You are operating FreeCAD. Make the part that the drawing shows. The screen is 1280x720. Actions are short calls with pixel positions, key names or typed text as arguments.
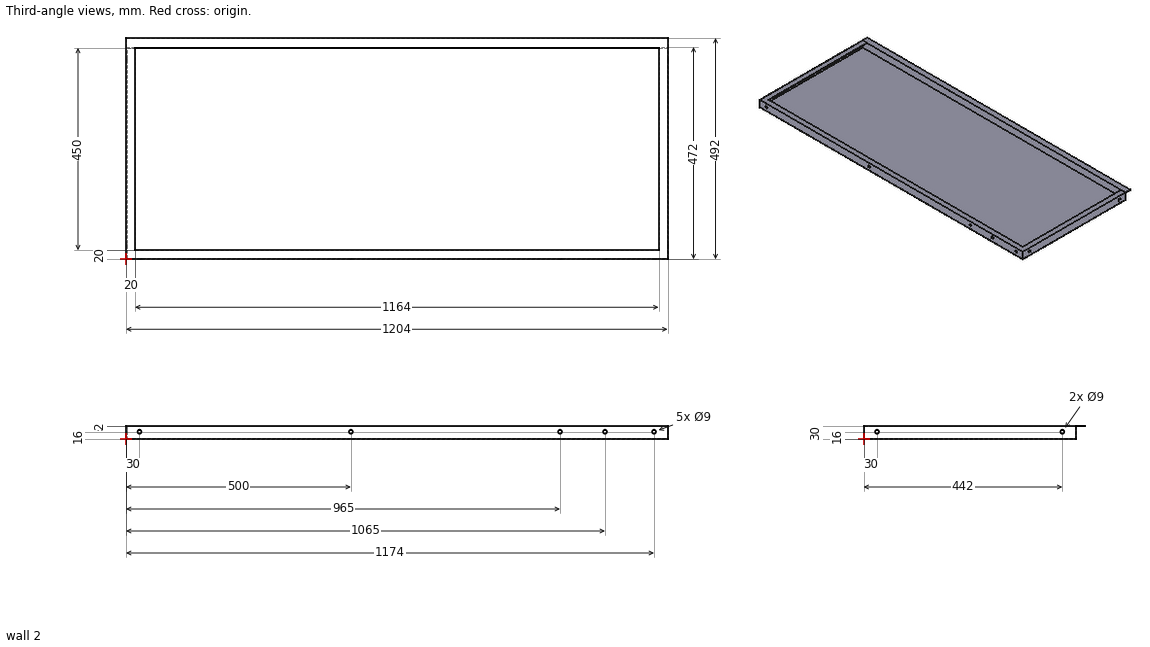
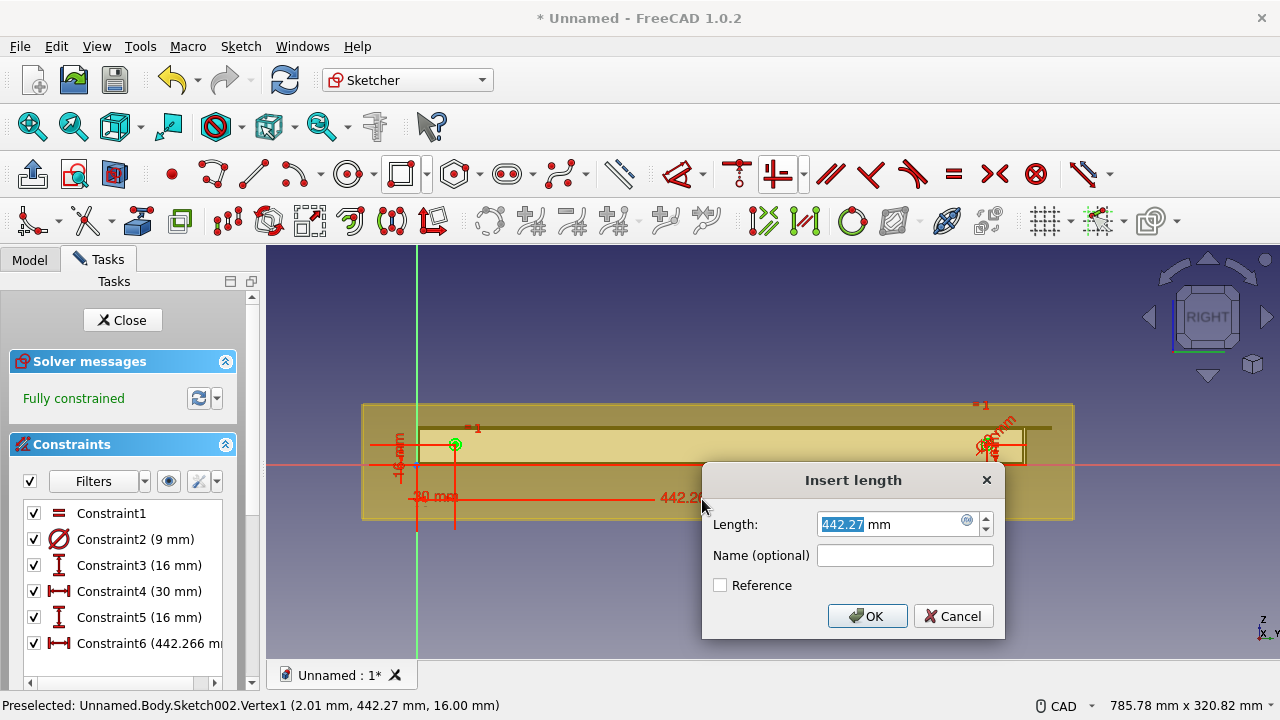
text(442)
key(Return)
key(Escape)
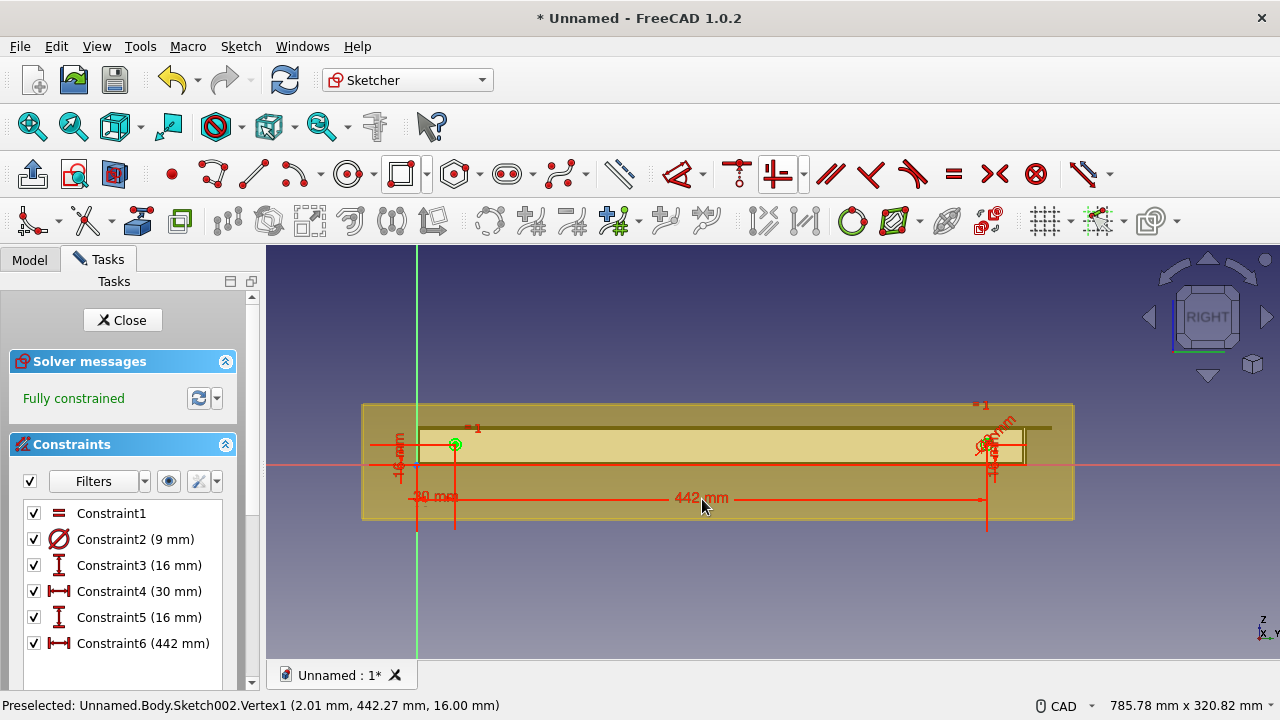
click(123, 320)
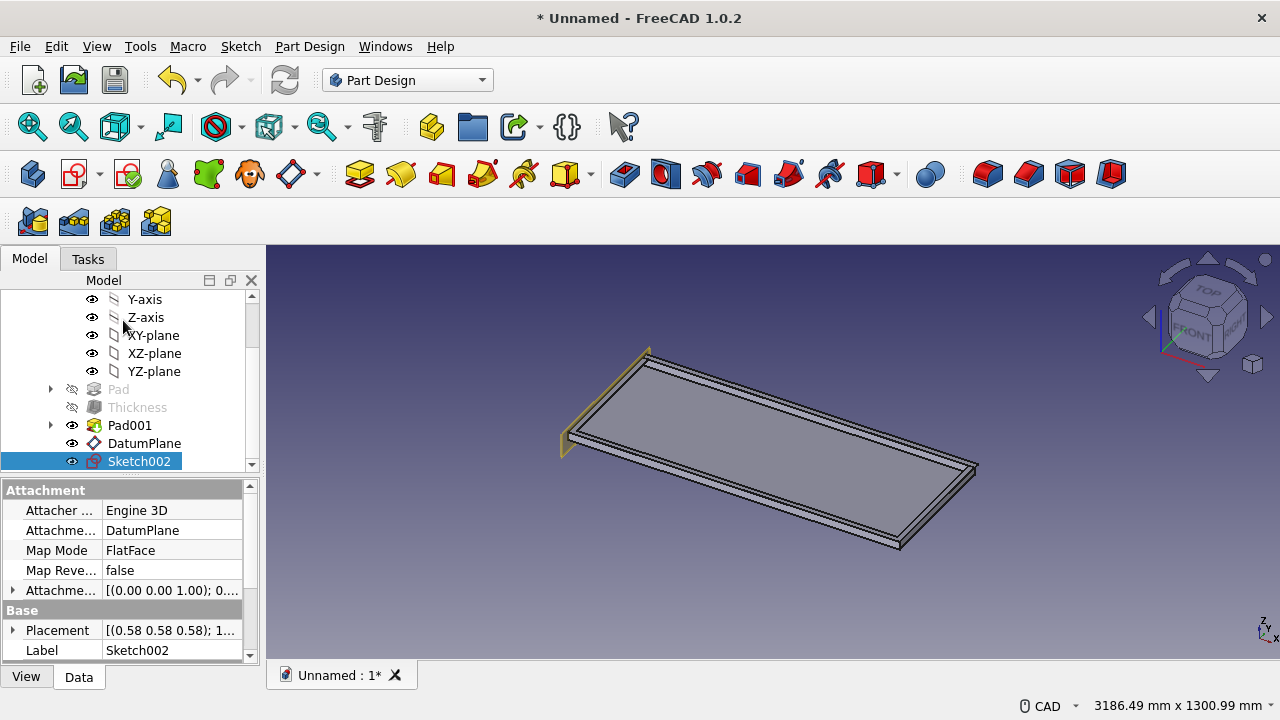
click(625, 174)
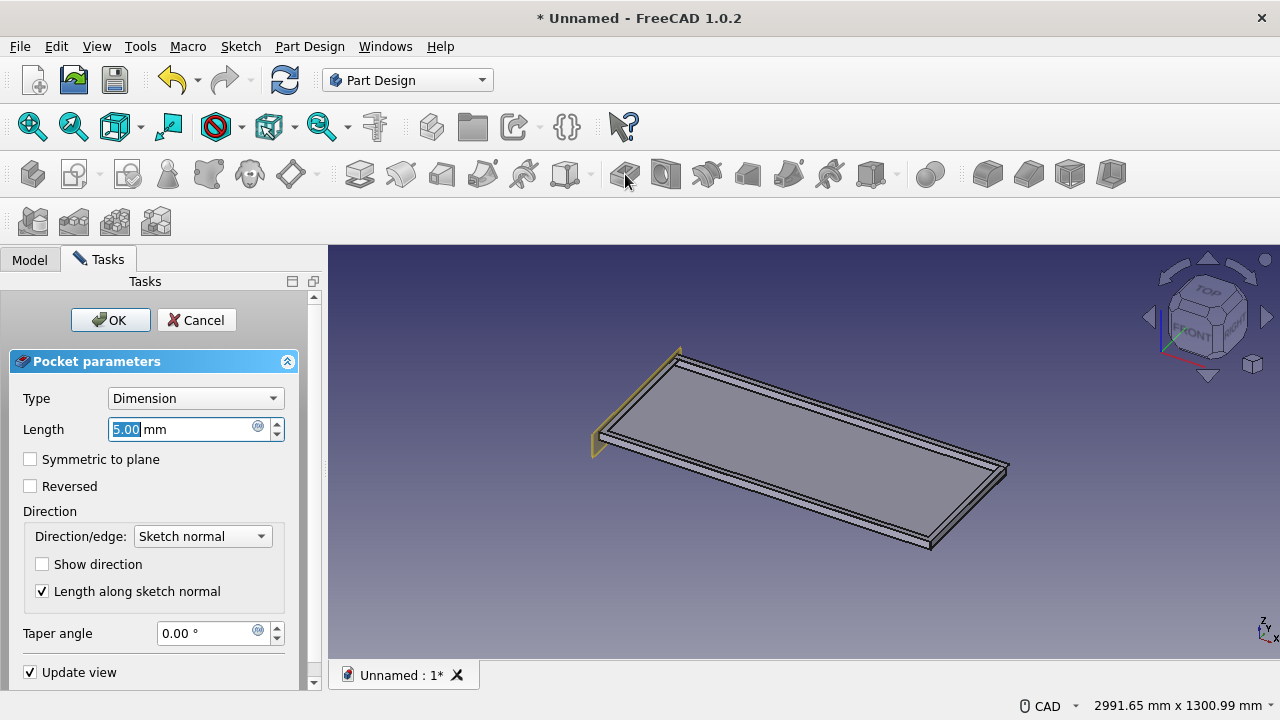
click(196, 398)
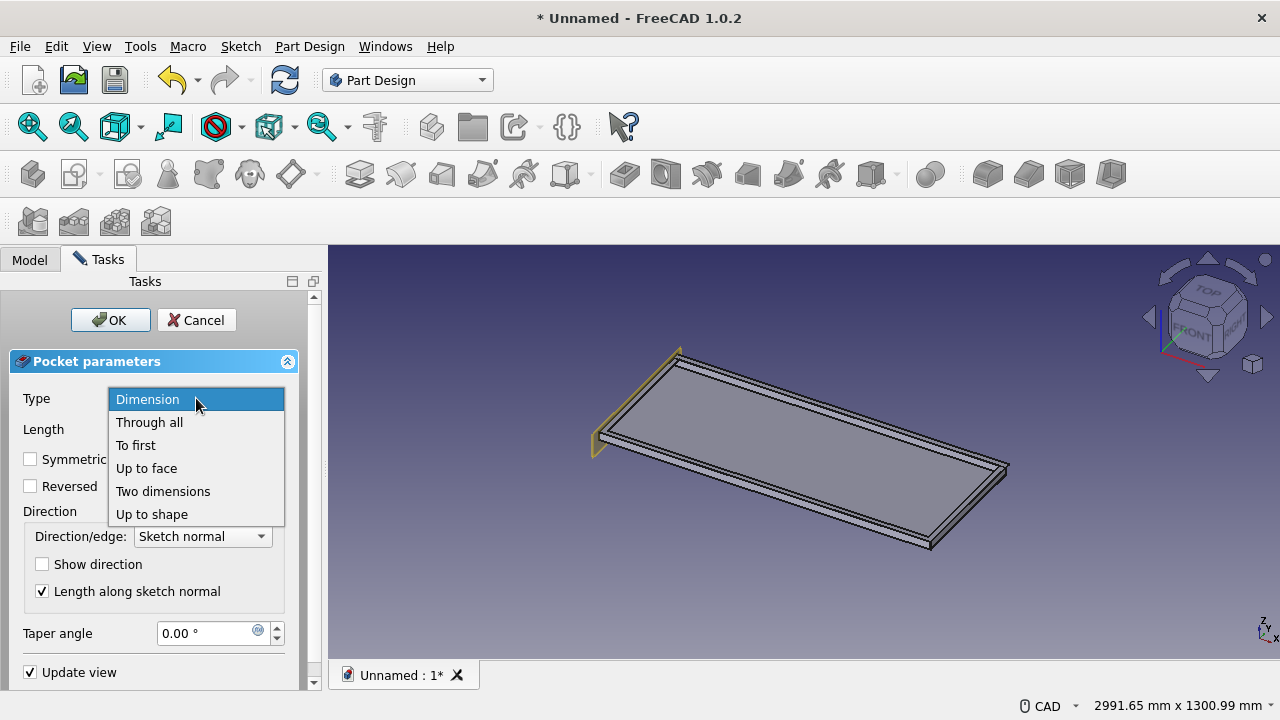
click(194, 492)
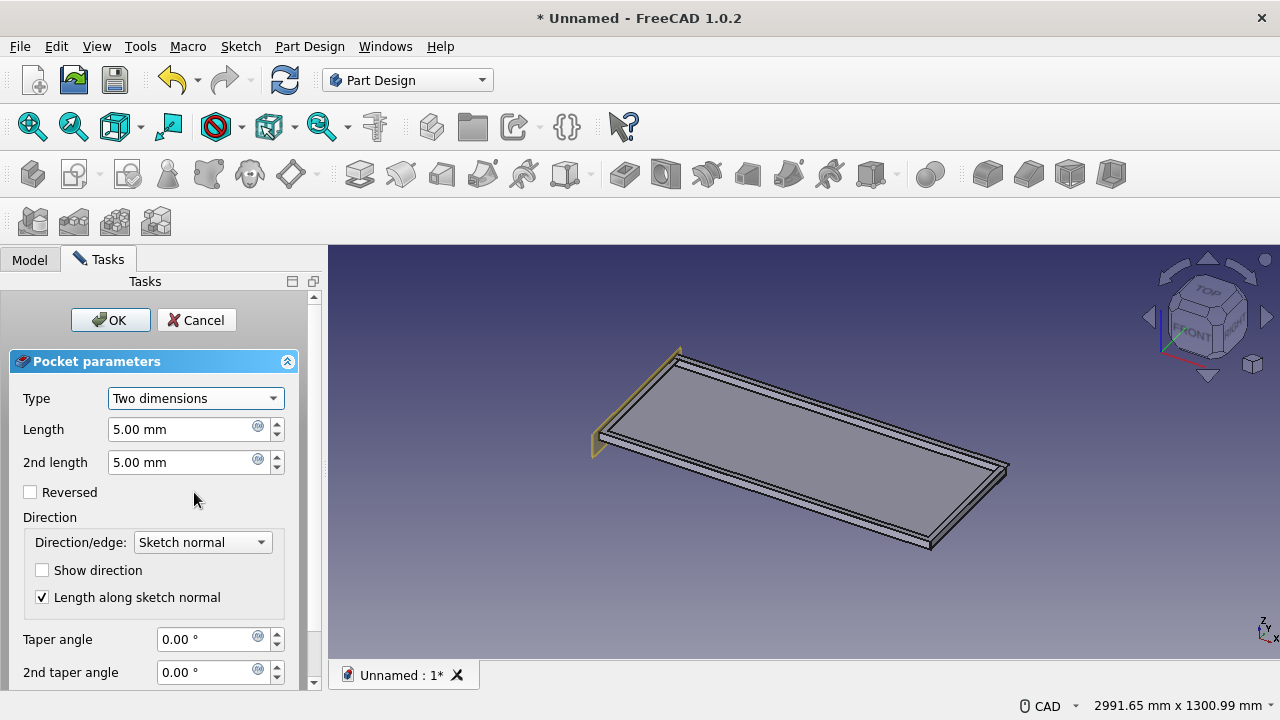
triple_click(190, 430)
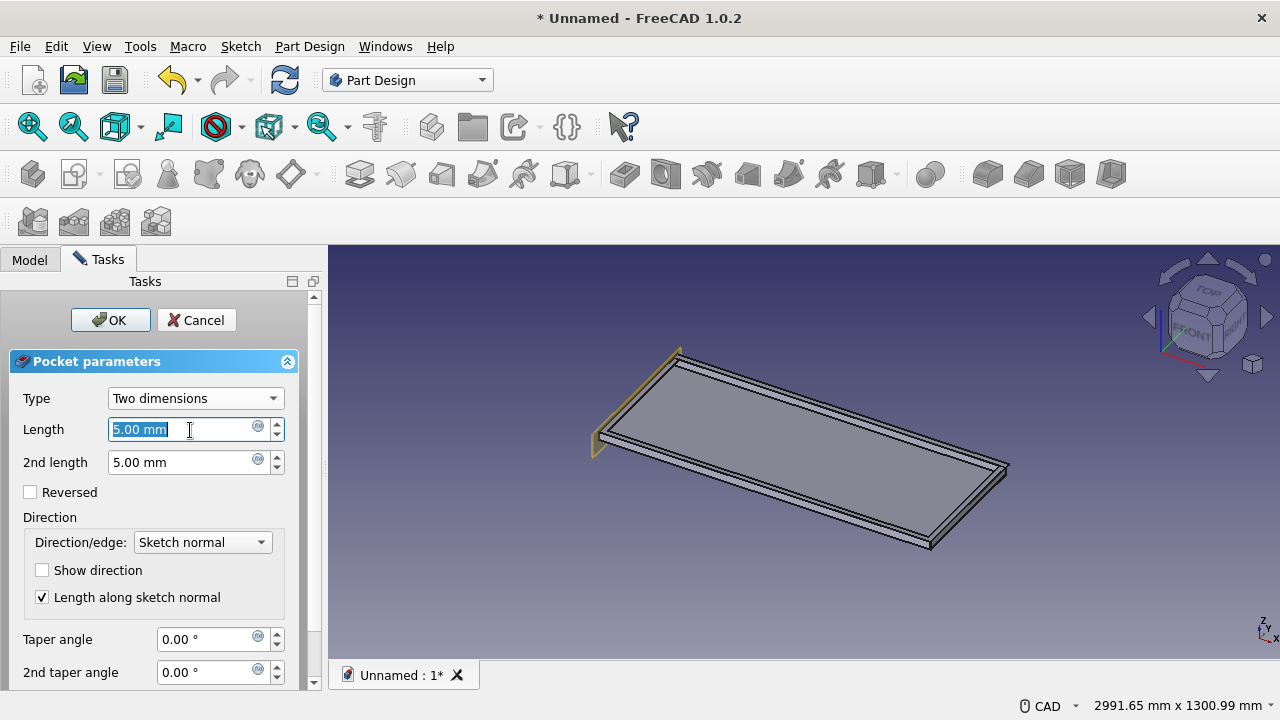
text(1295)
key(Tab)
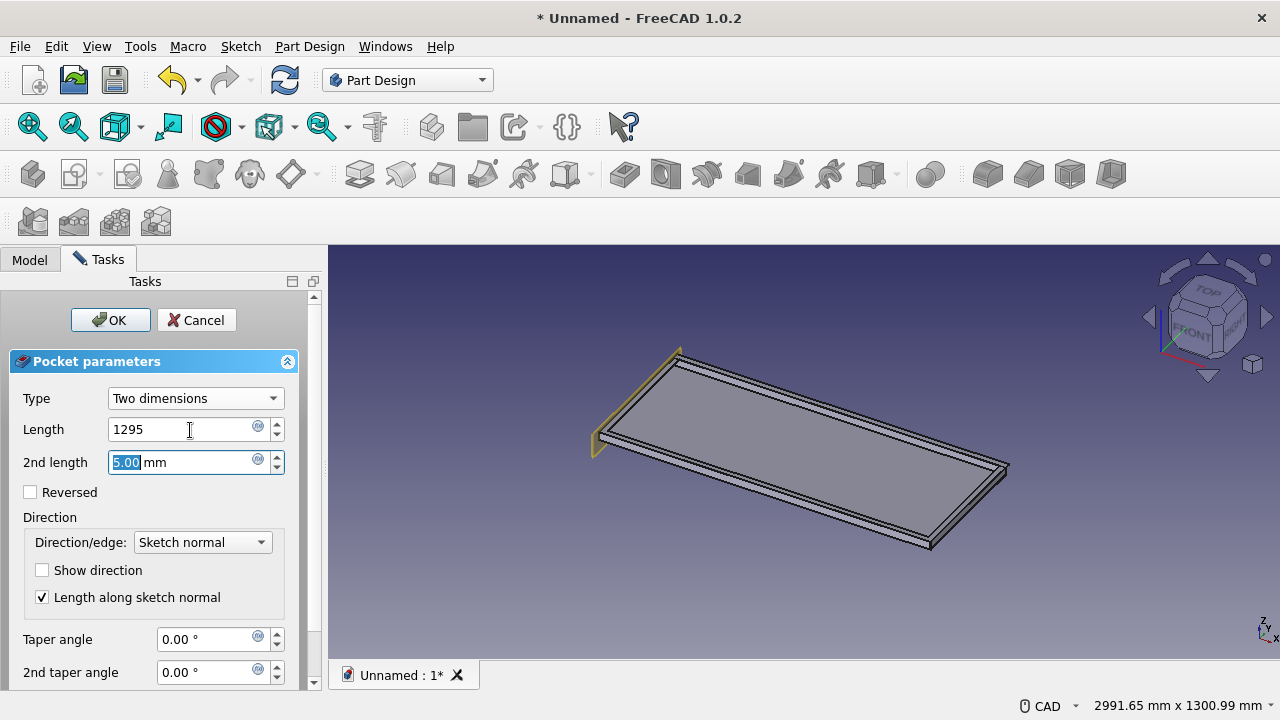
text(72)
key(Tab)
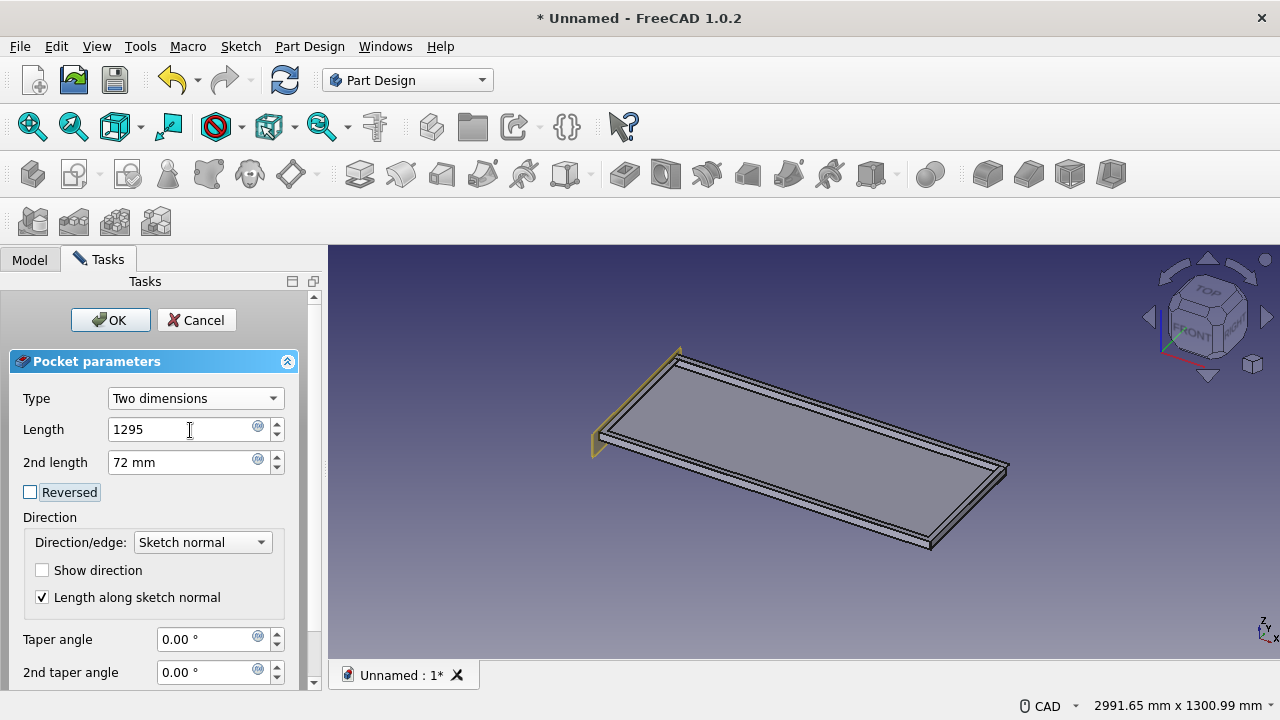
click(31, 492)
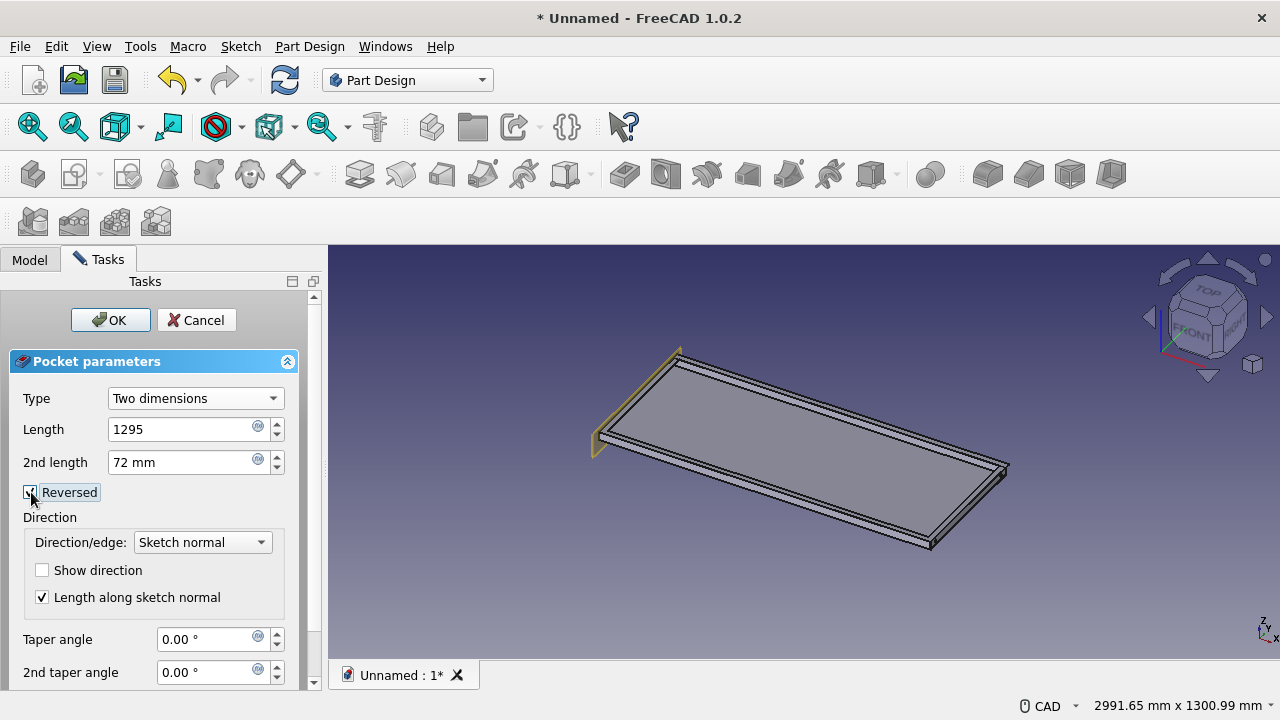
click(111, 320)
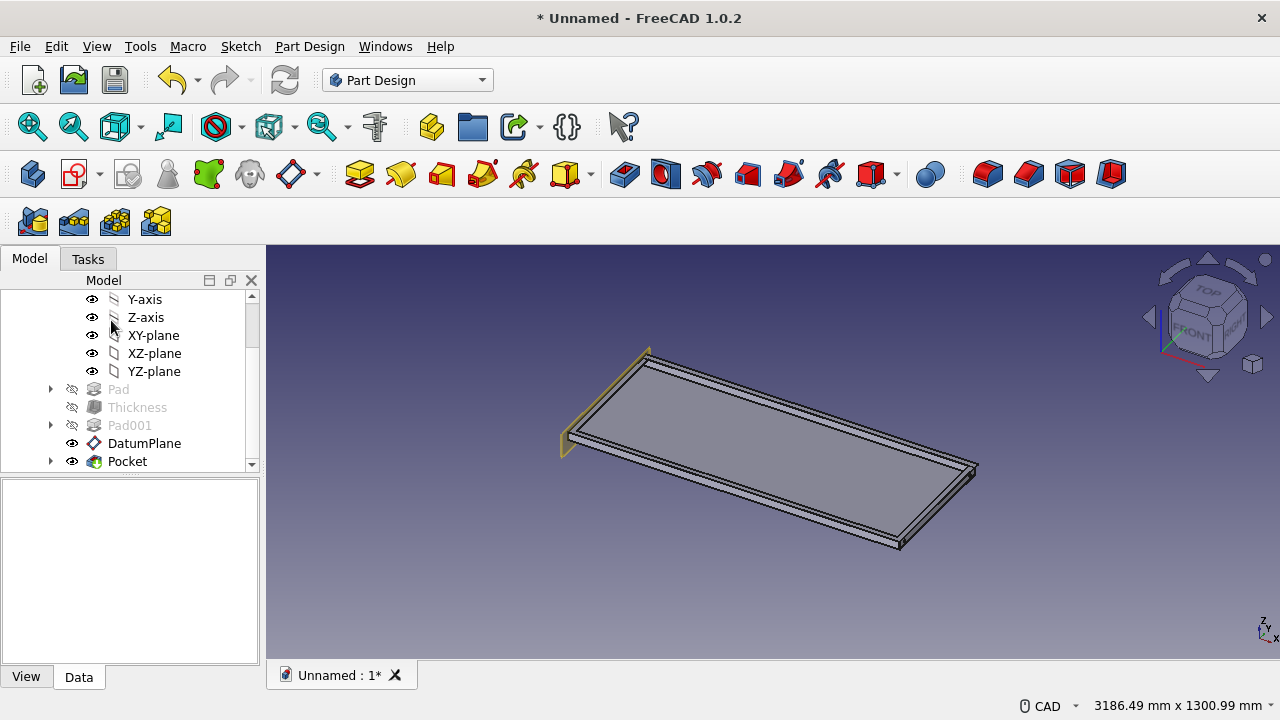
click(117, 443)
key(space)